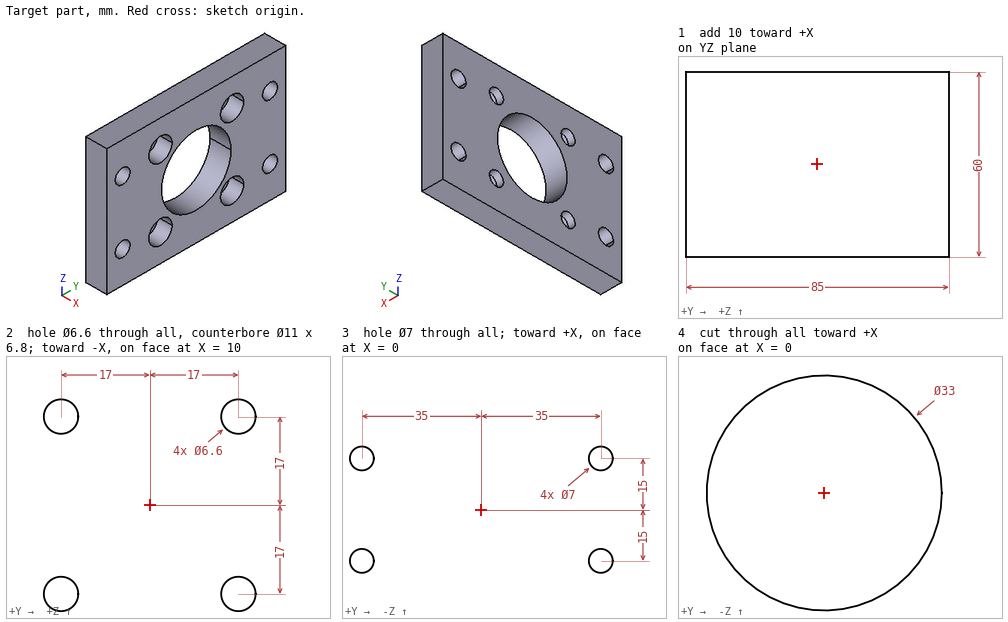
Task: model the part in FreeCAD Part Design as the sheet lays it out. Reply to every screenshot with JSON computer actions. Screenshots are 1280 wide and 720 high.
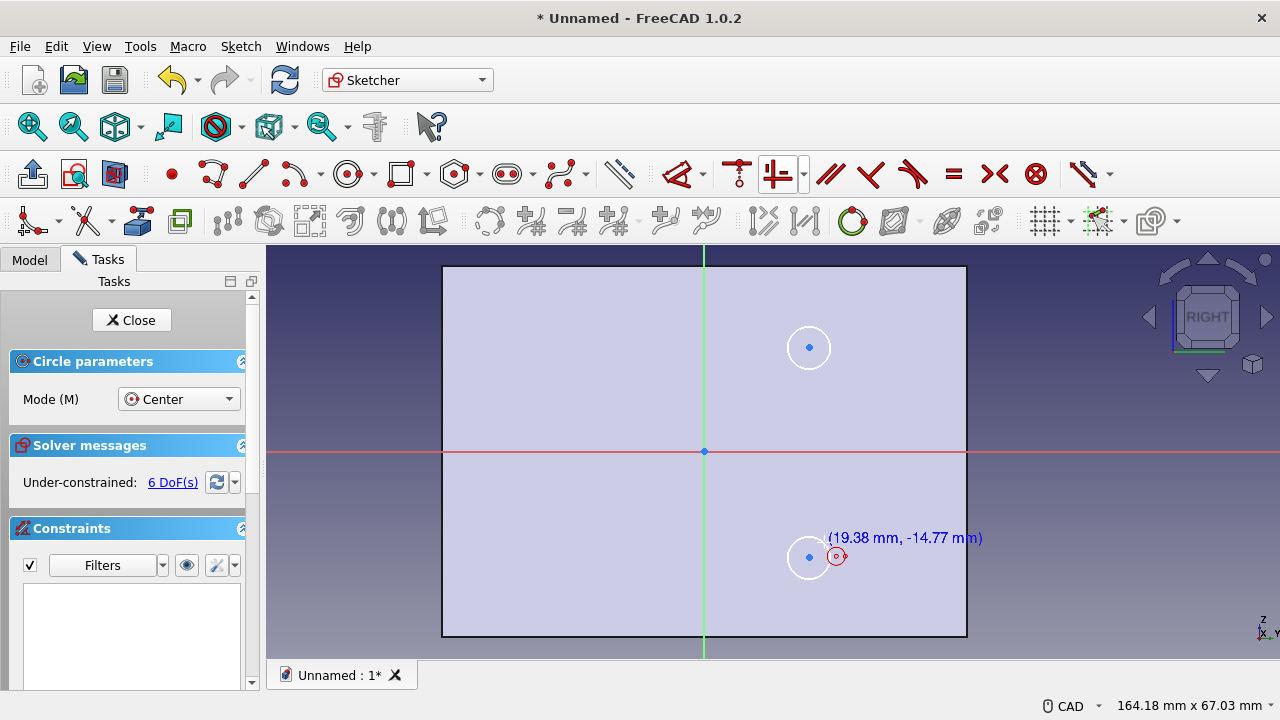
{"action": "left_click", "coordinate": [599, 347]}
{"action": "left_click", "coordinate": [614, 332]}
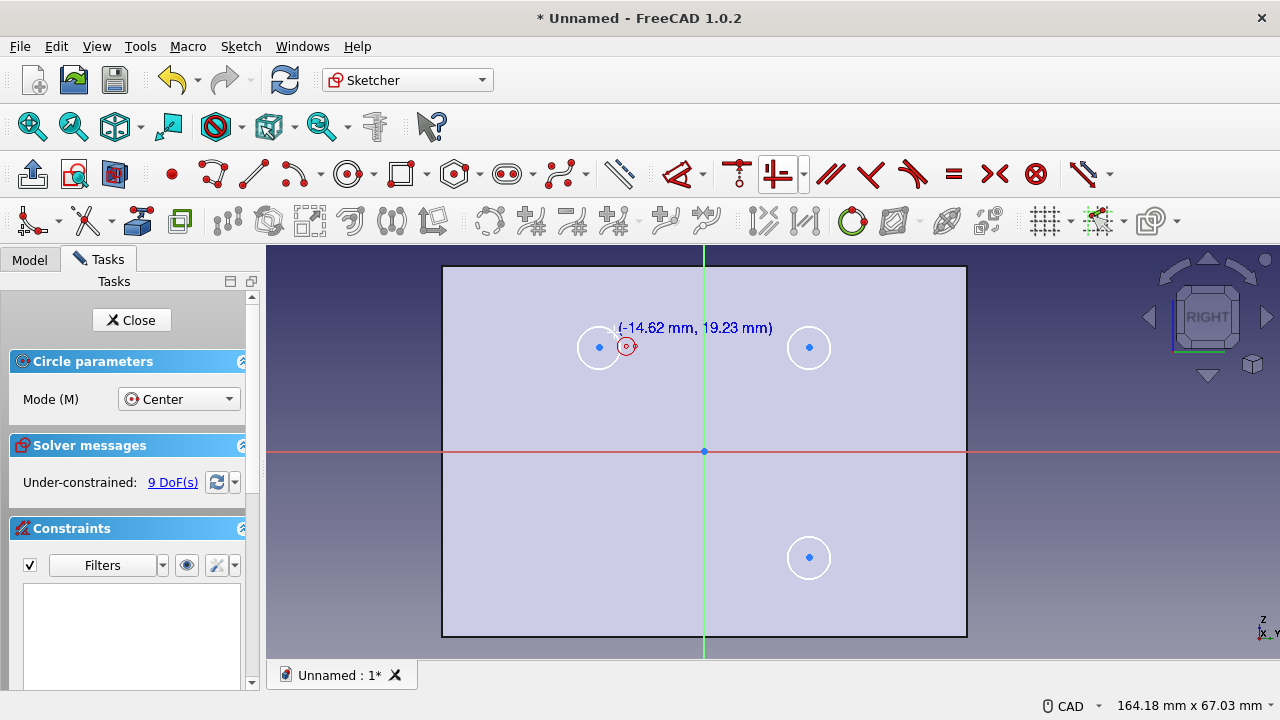
{"action": "left_click", "coordinate": [599, 557]}
{"action": "left_click", "coordinate": [614, 542]}
{"action": "key", "text": "Escape"}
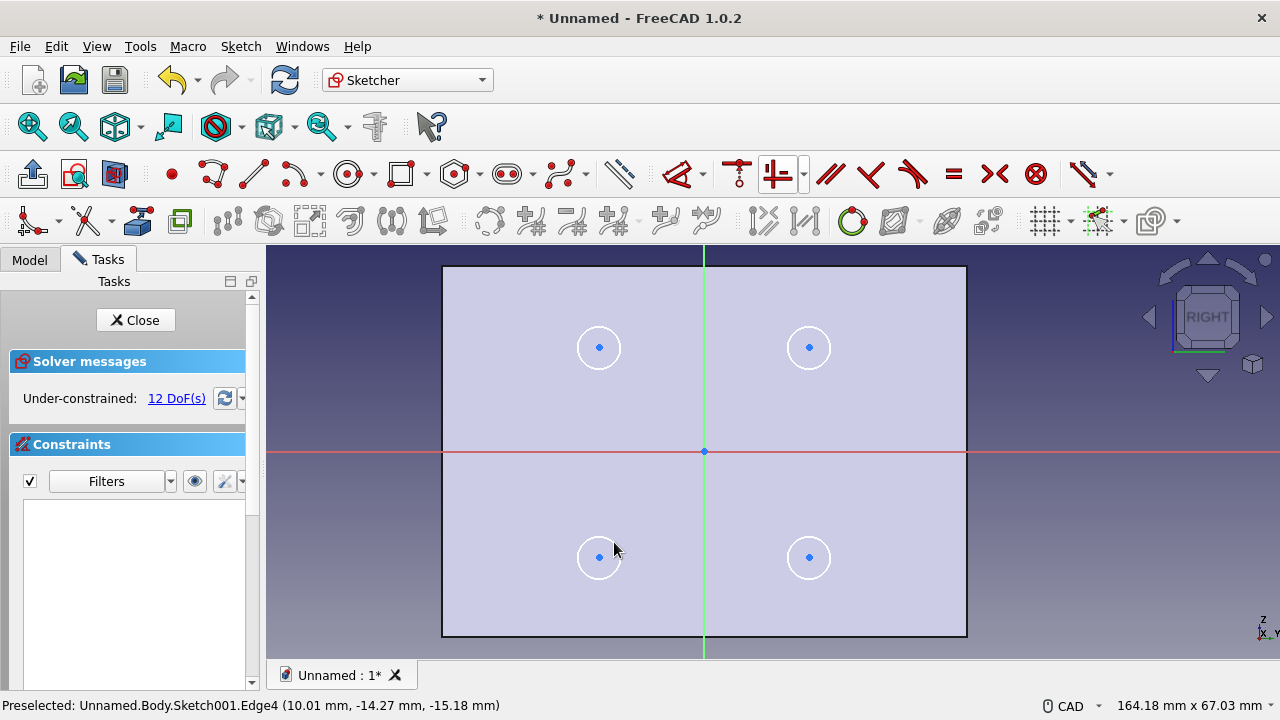
{"action": "left_click", "coordinate": [824, 333]}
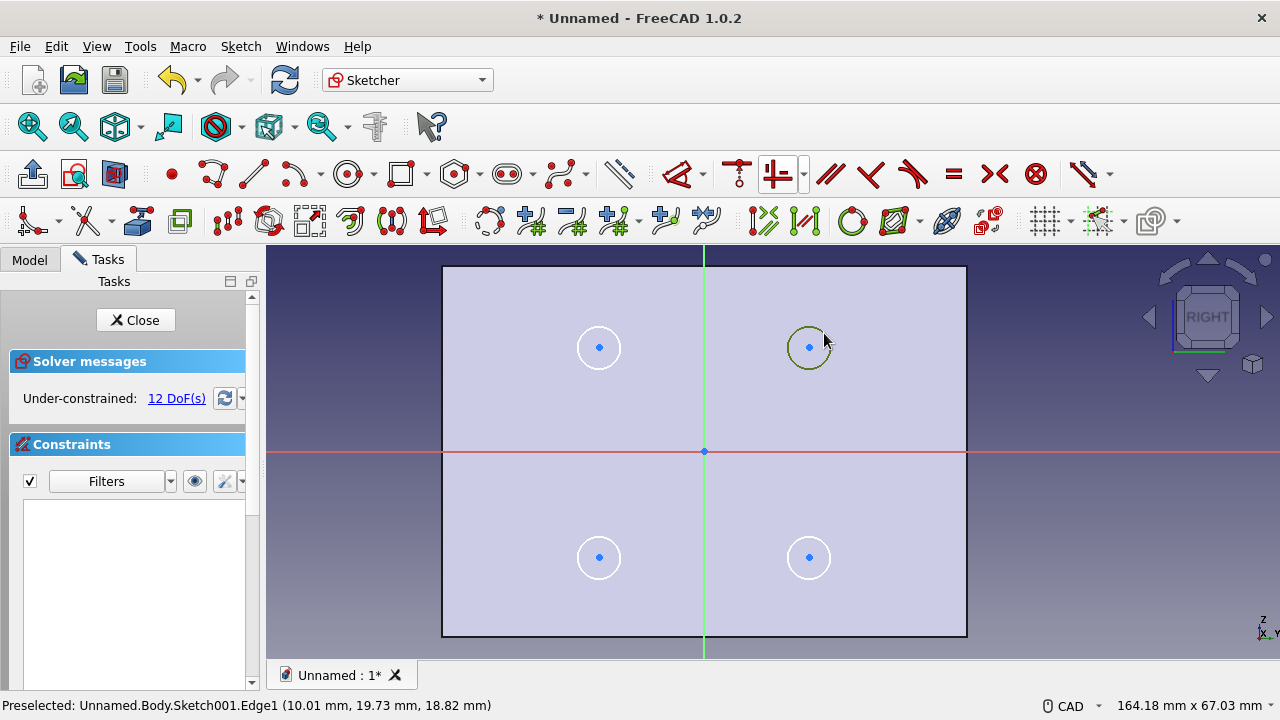
{"action": "left_click", "coordinate": [824, 543]}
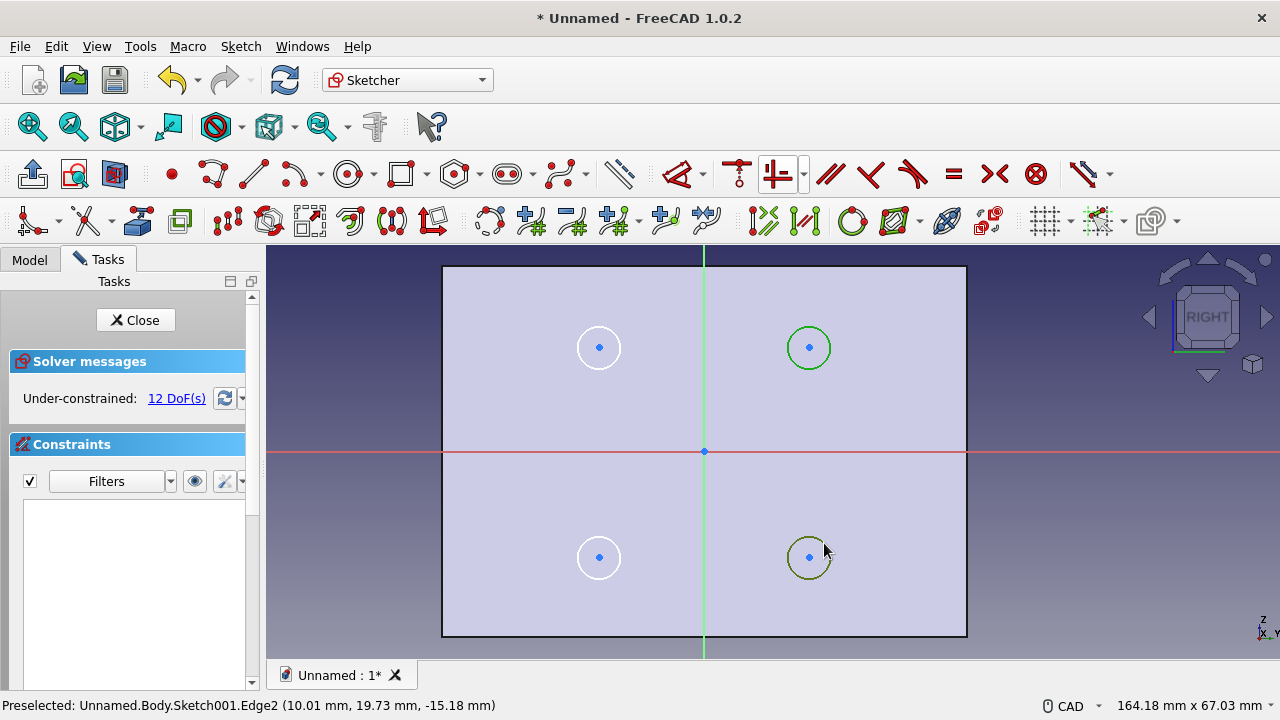
{"action": "left_click", "coordinate": [614, 333]}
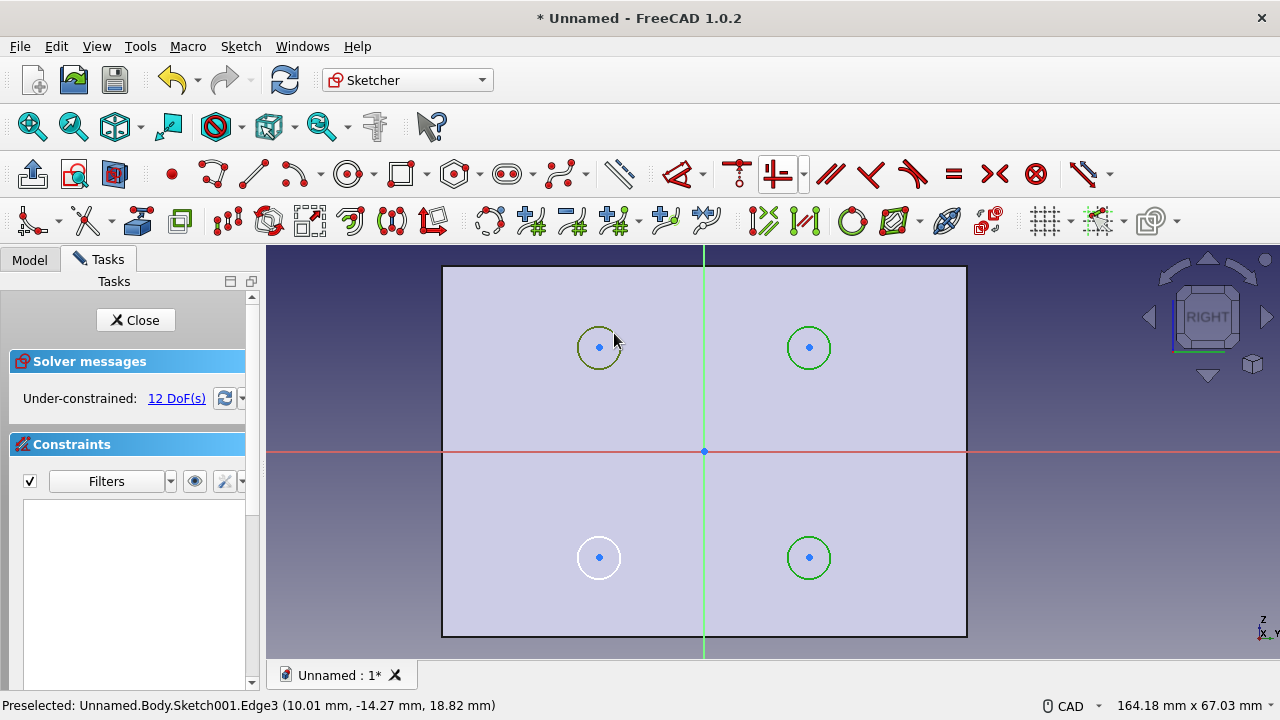
{"action": "left_click", "coordinate": [614, 543]}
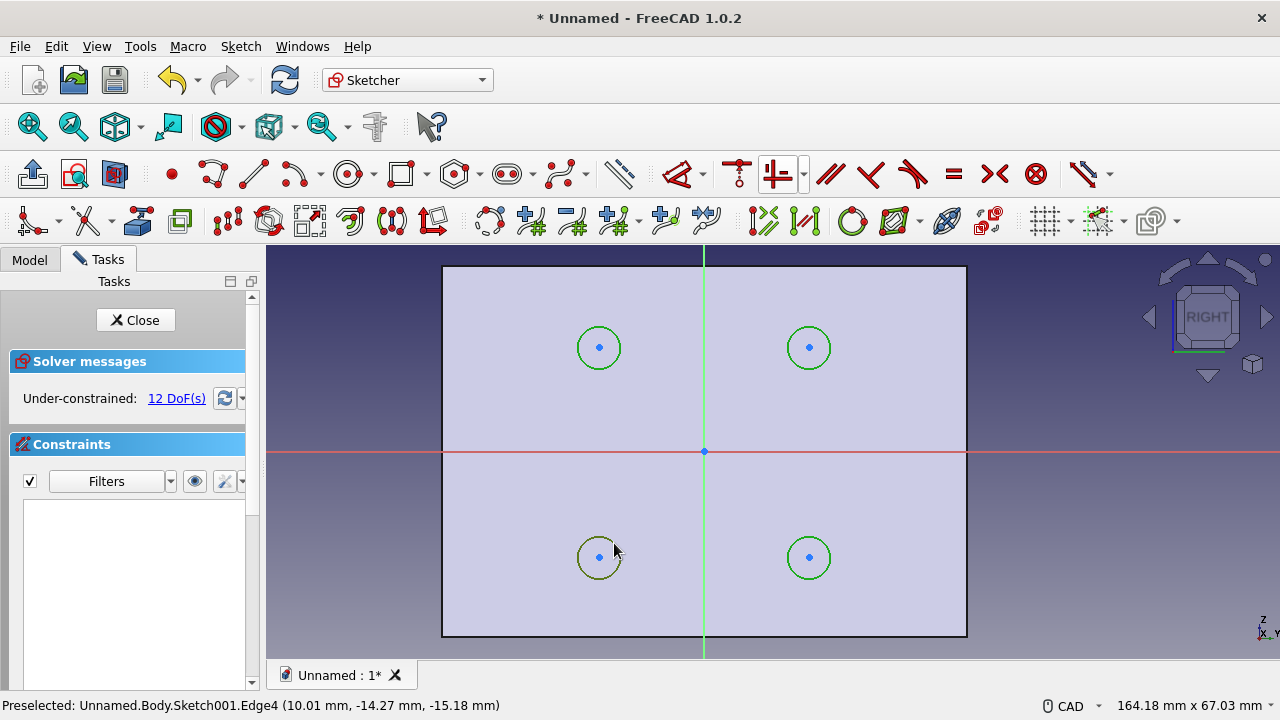
{"action": "left_click", "coordinate": [954, 174]}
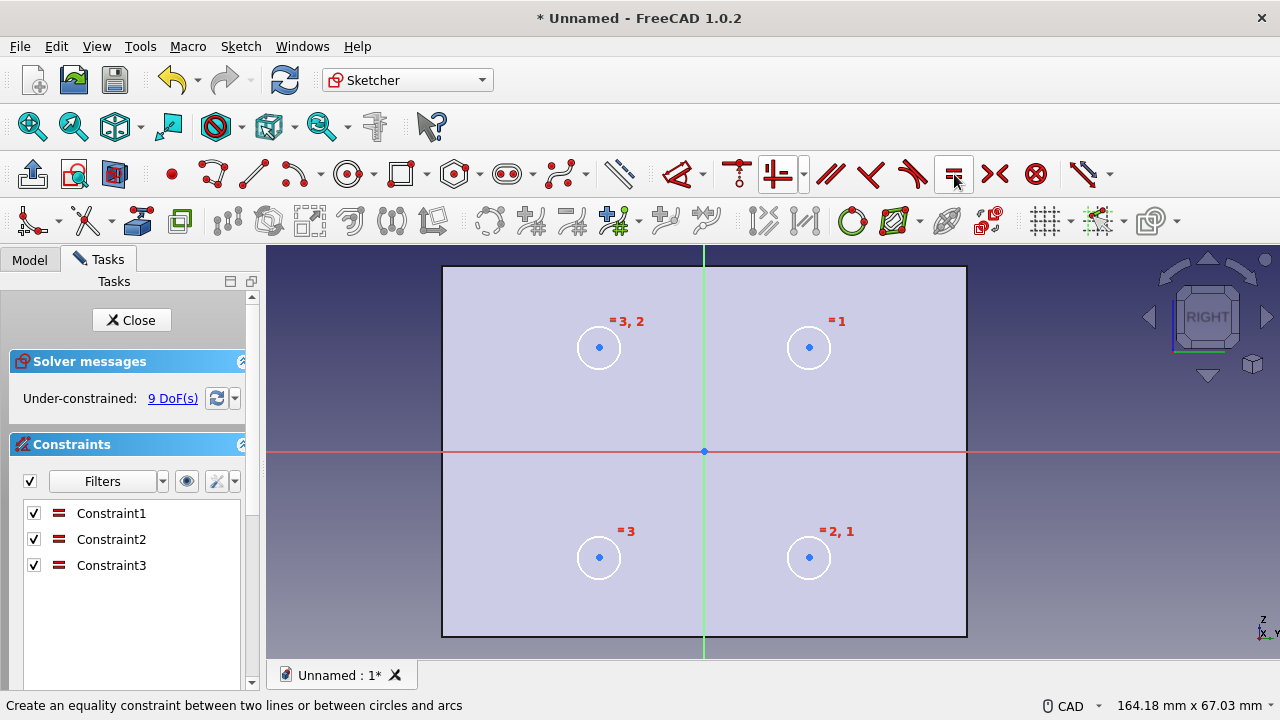
{"action": "left_click", "coordinate": [809, 348]}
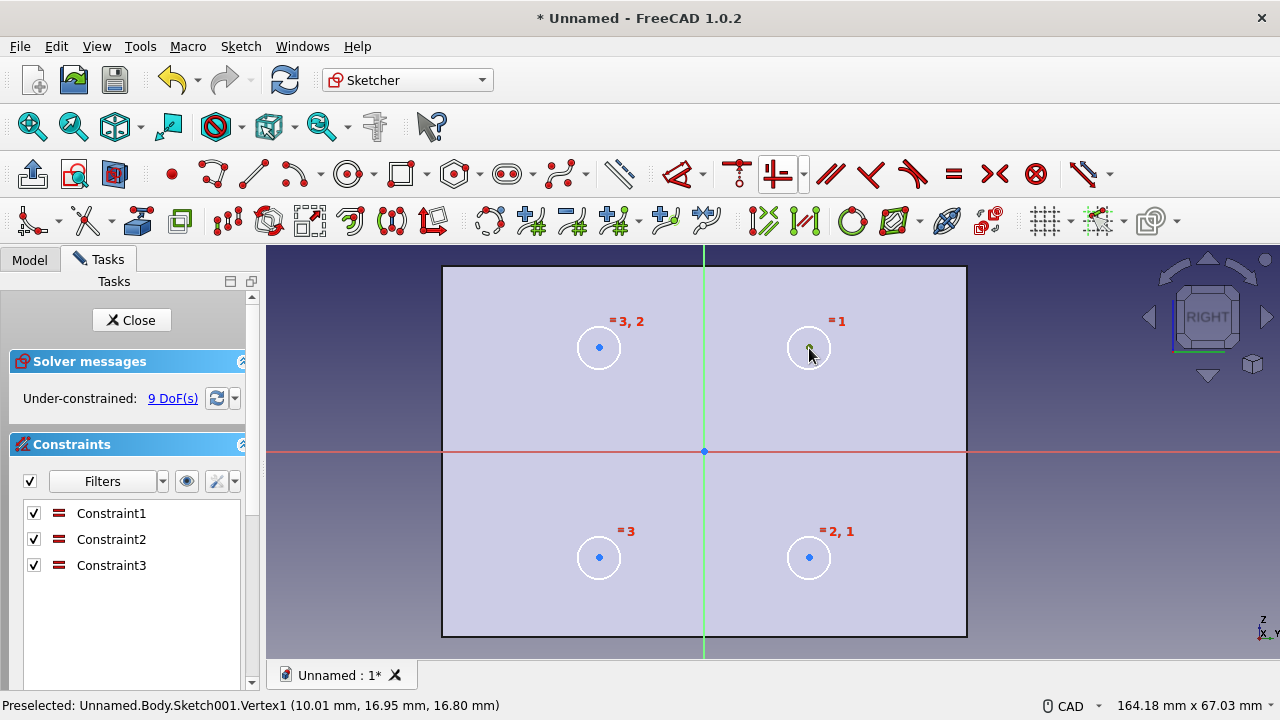
{"action": "left_click", "coordinate": [809, 558]}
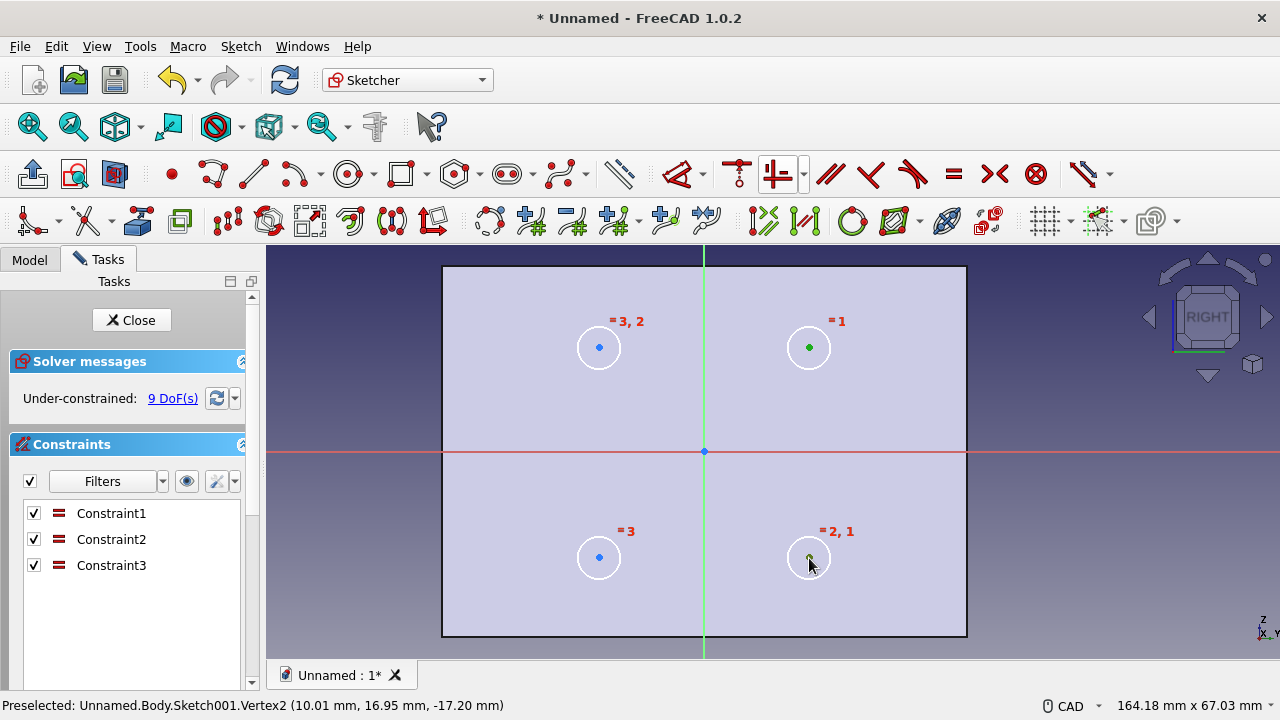
{"action": "key", "text": "v"}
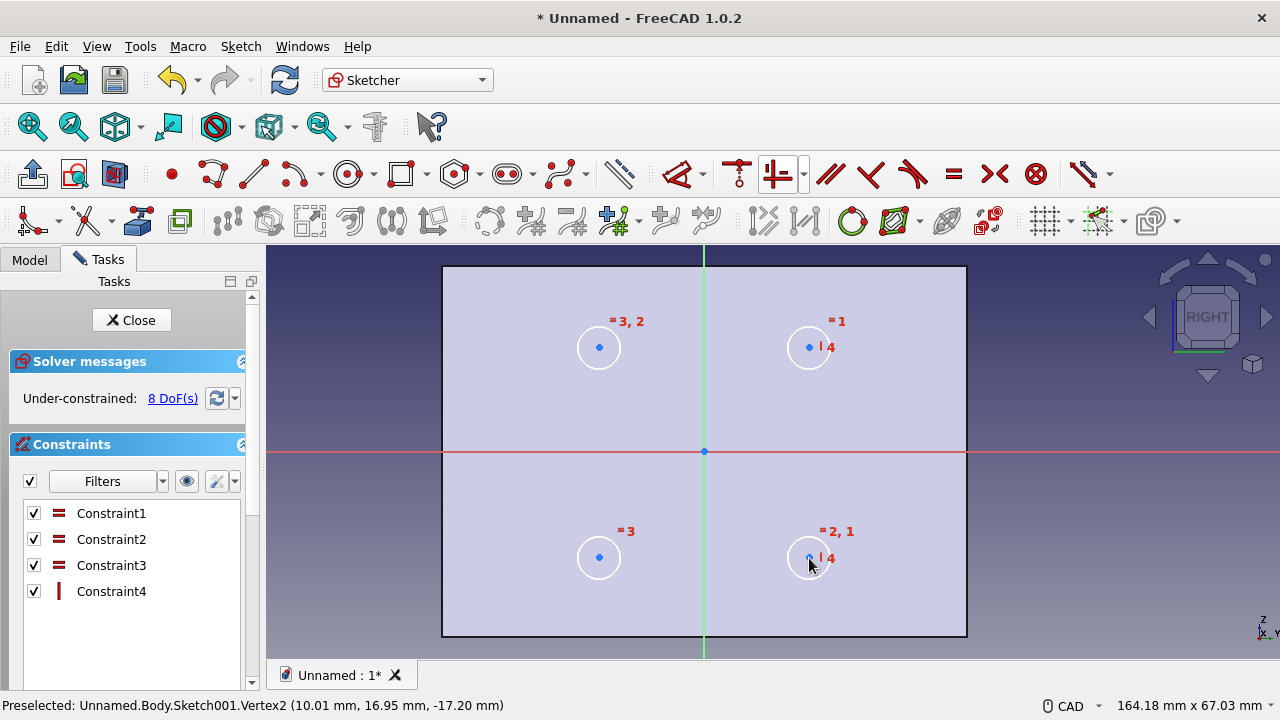
{"action": "left_click", "coordinate": [809, 348]}